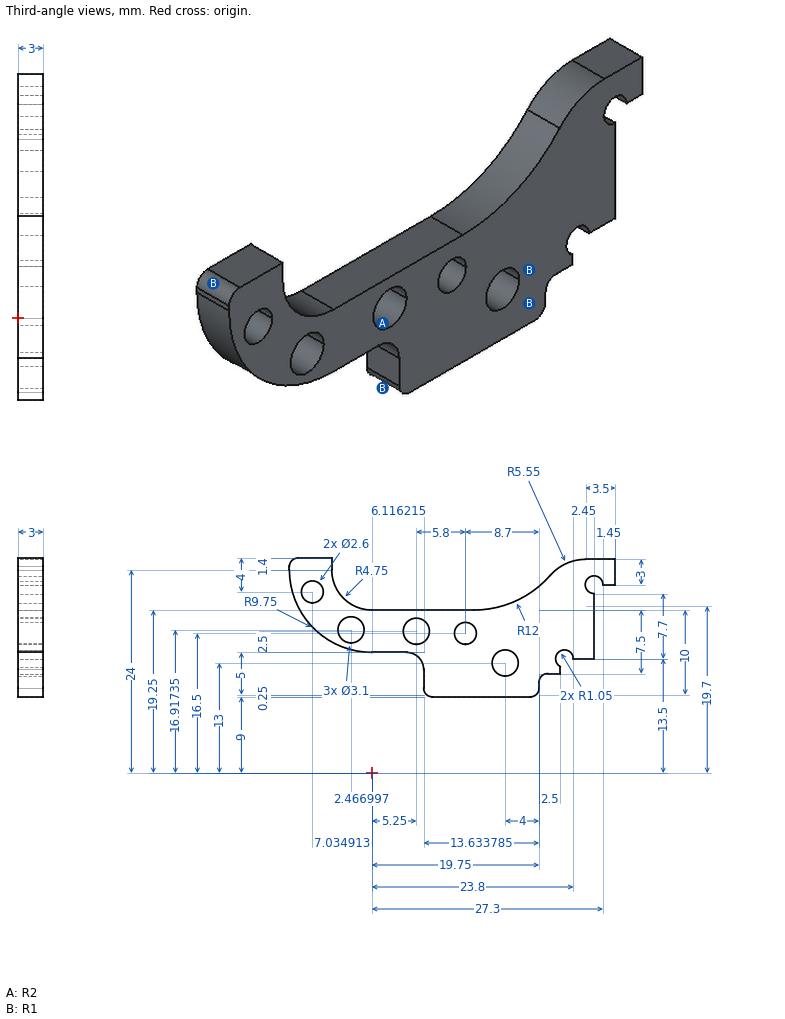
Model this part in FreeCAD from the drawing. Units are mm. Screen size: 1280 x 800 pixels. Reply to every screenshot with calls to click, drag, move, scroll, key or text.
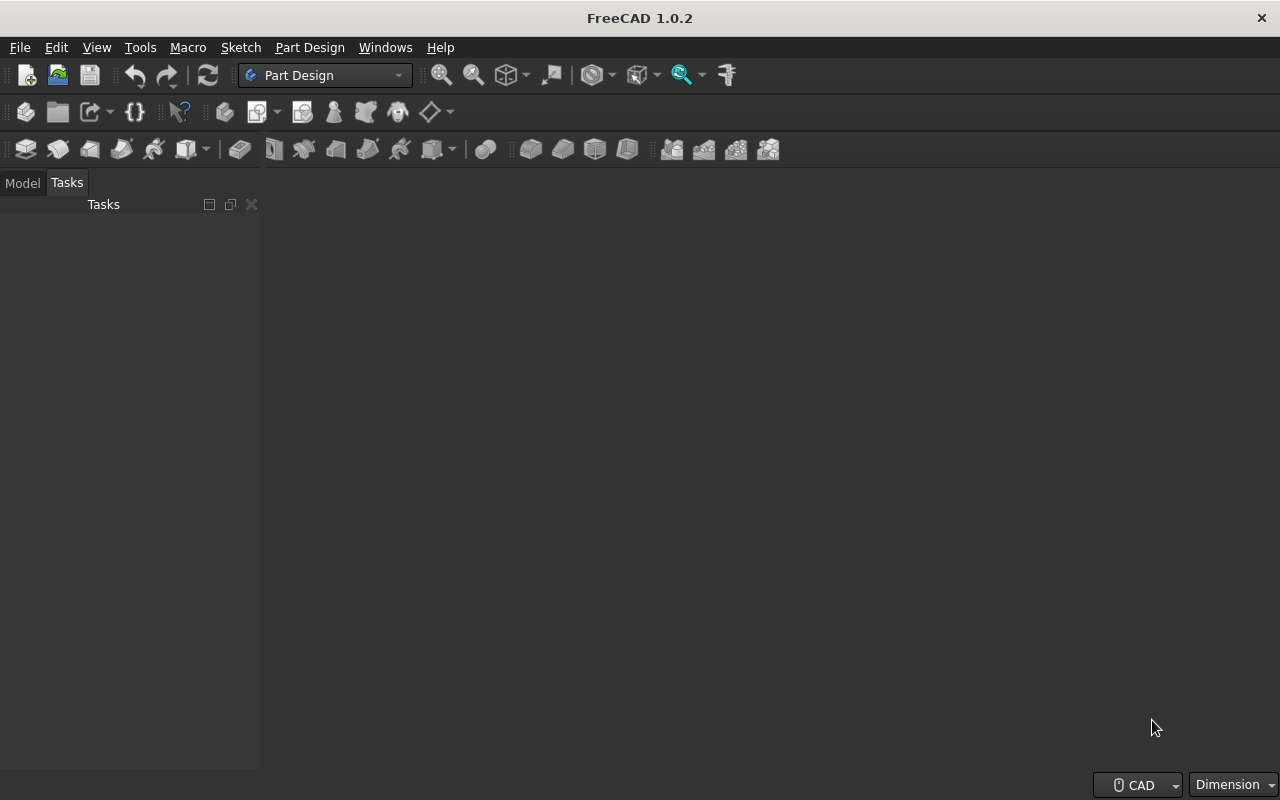
key(ctrl+n)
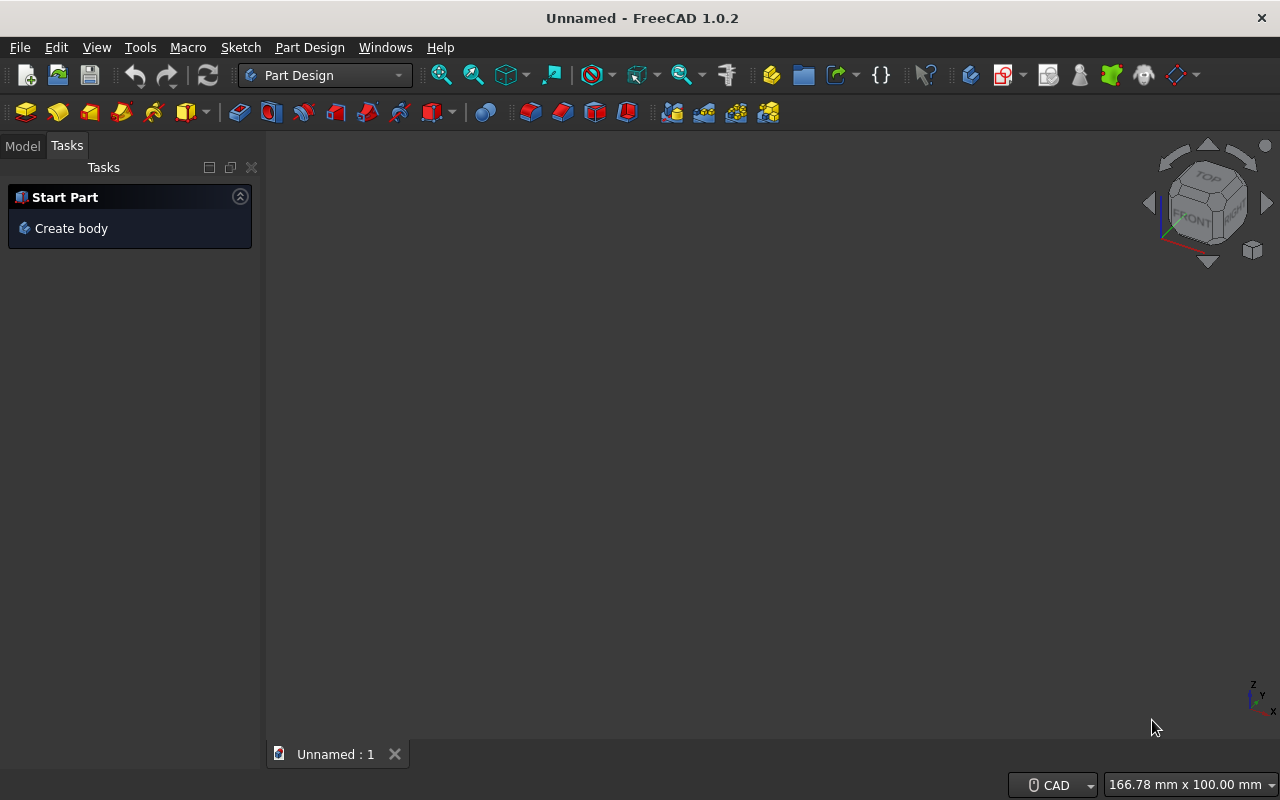
click(1004, 76)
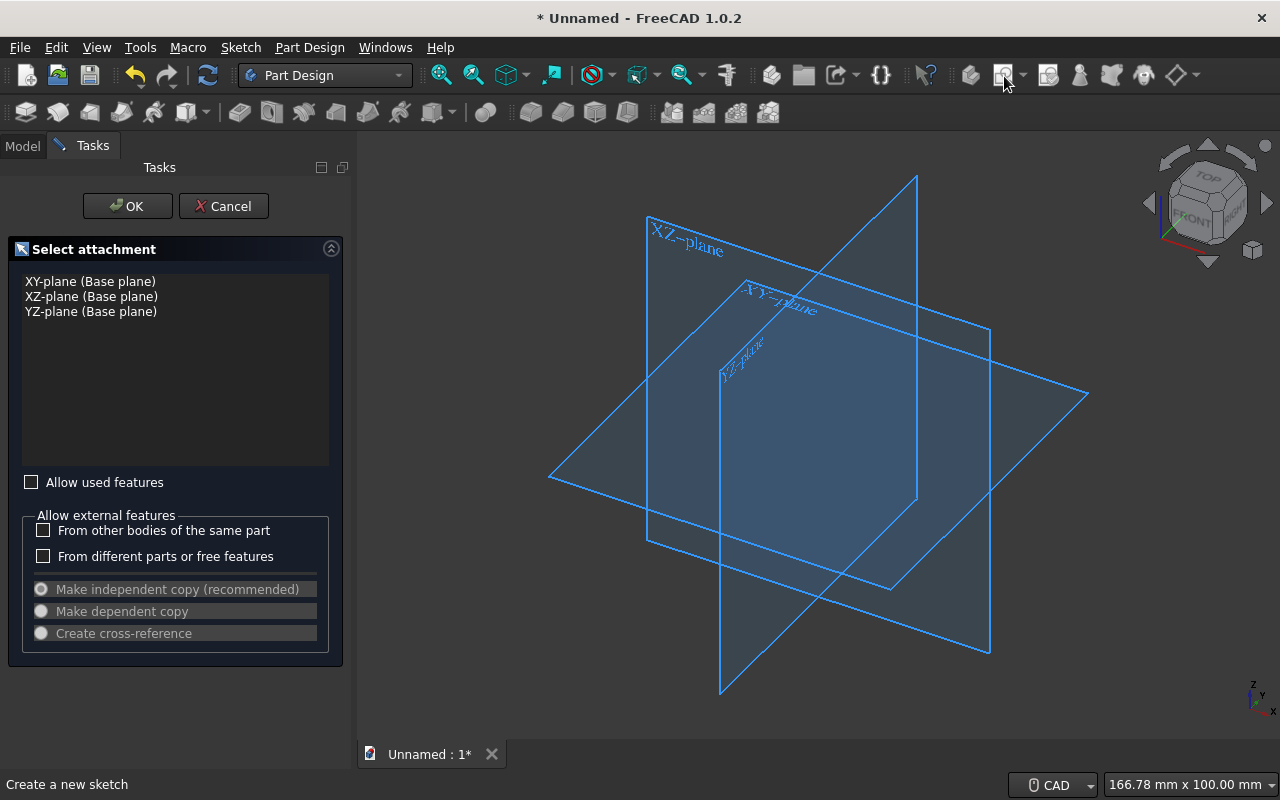
click(82, 312)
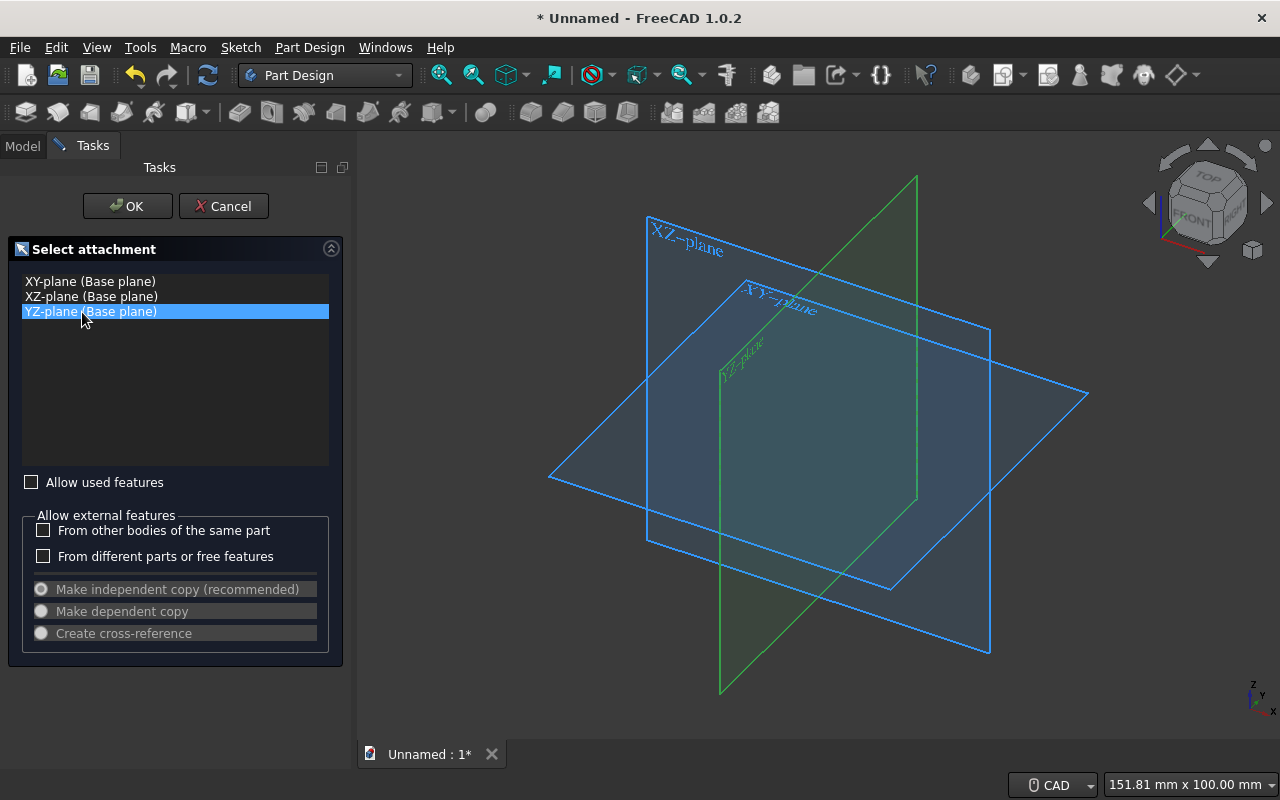
click(128, 206)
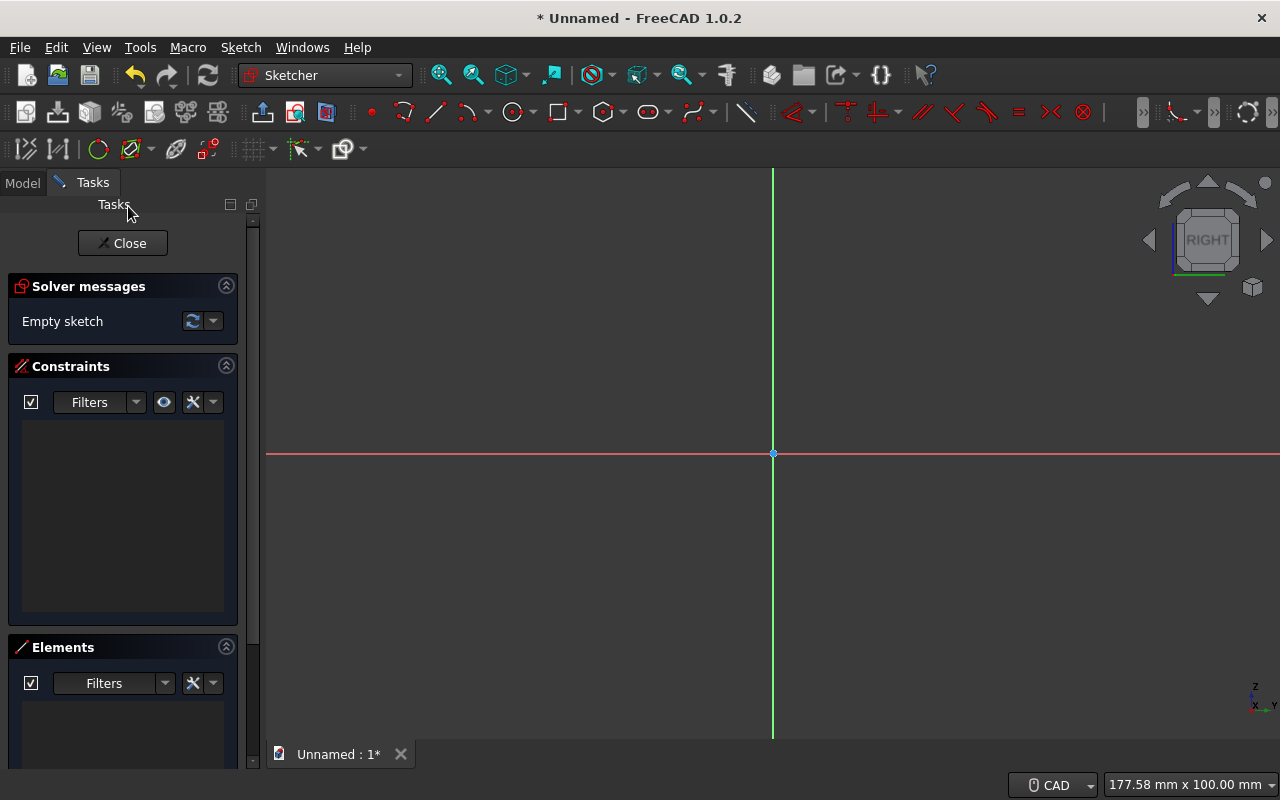
scroll(858, 339, up, 5)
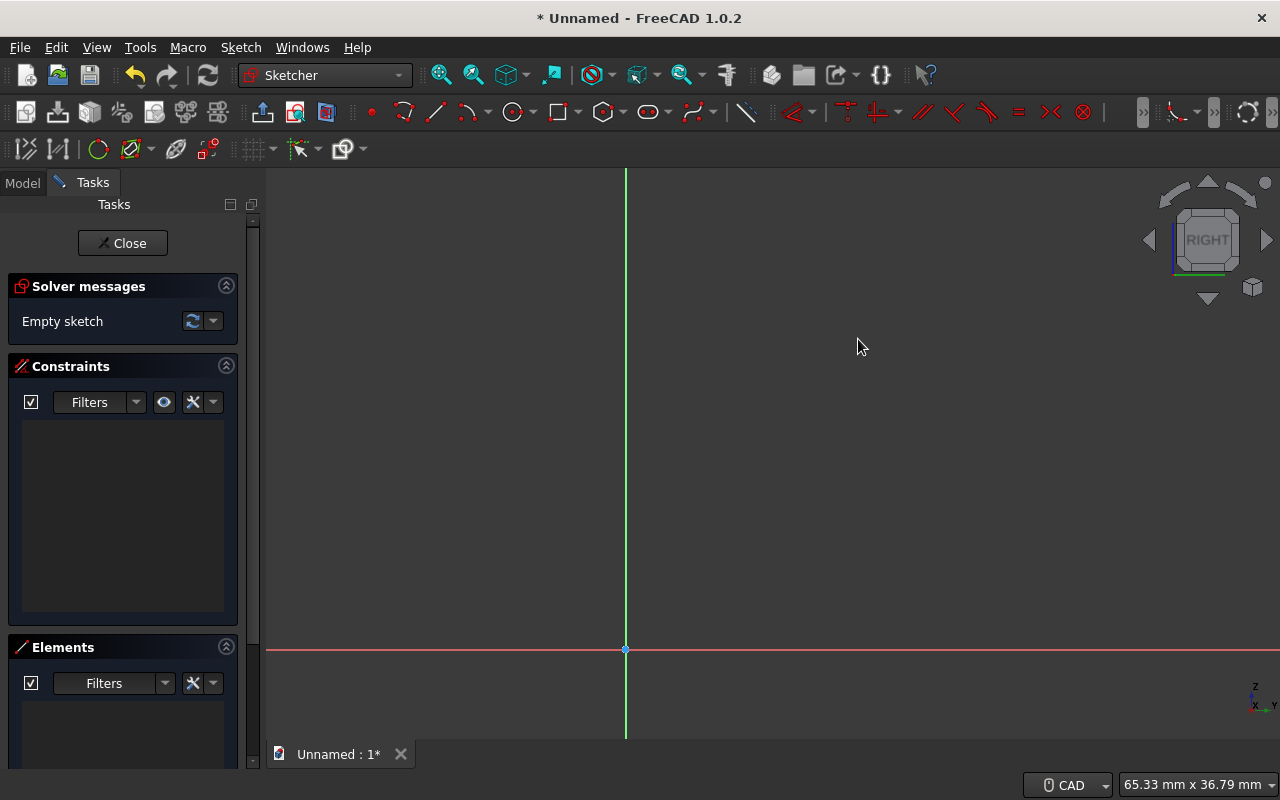
key(g)
key(m)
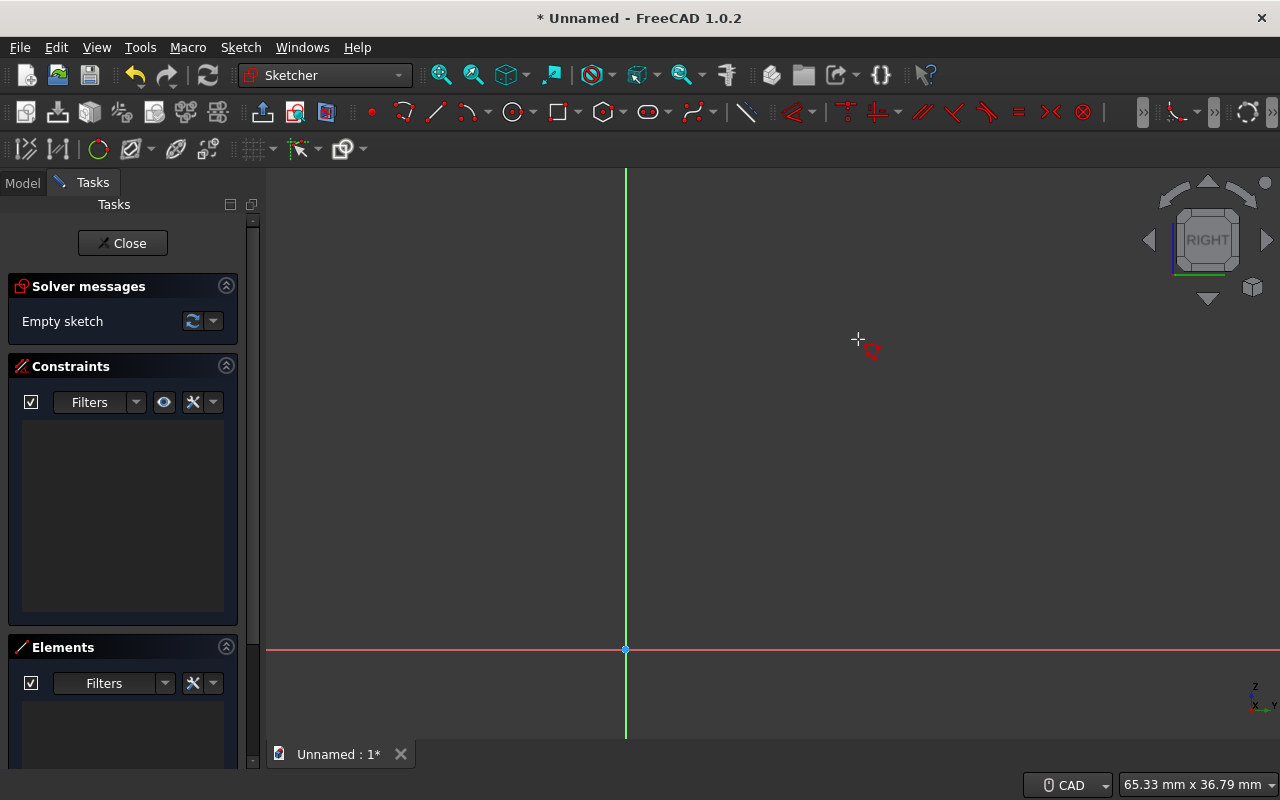
click(552, 277)
click(552, 255)
click(475, 255)
click(475, 277)
right_click(475, 277)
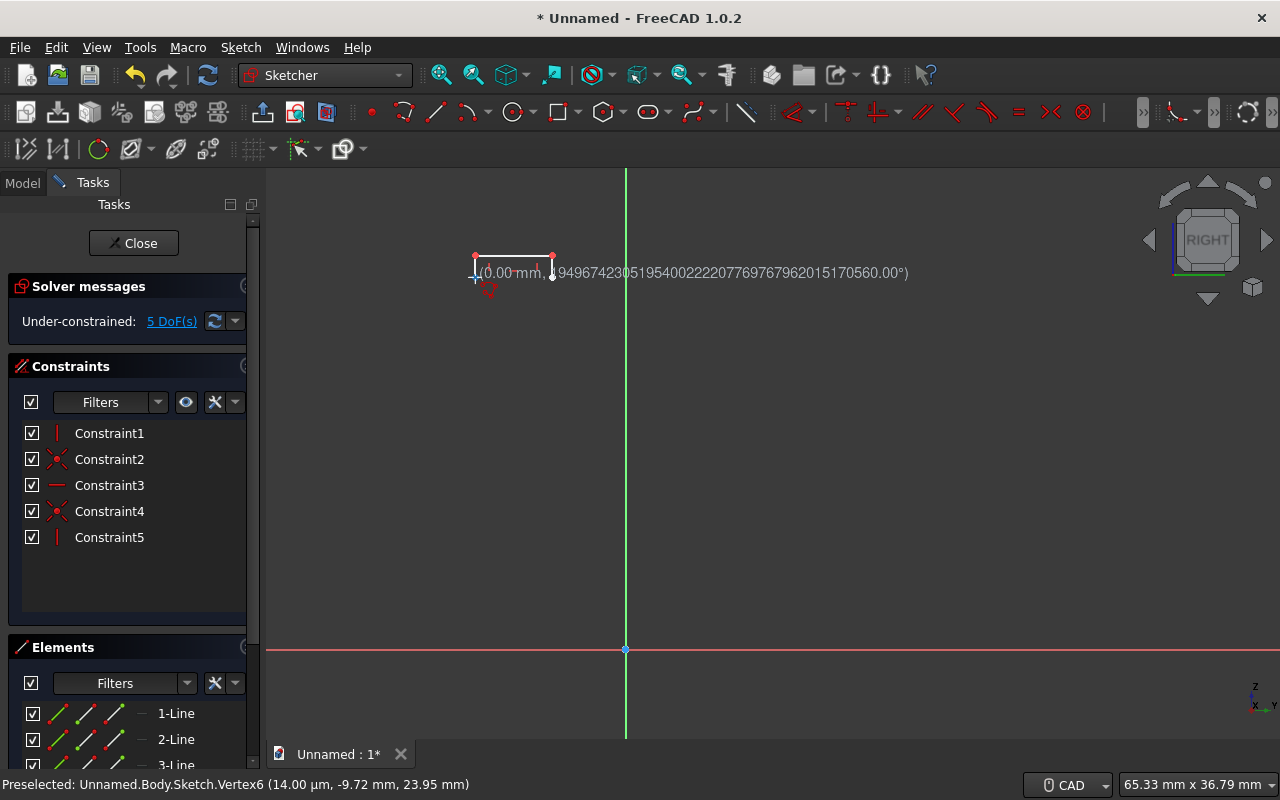
click(626, 429)
click(721, 429)
click(721, 506)
click(932, 506)
click(932, 351)
click(626, 351)
right_click(626, 351)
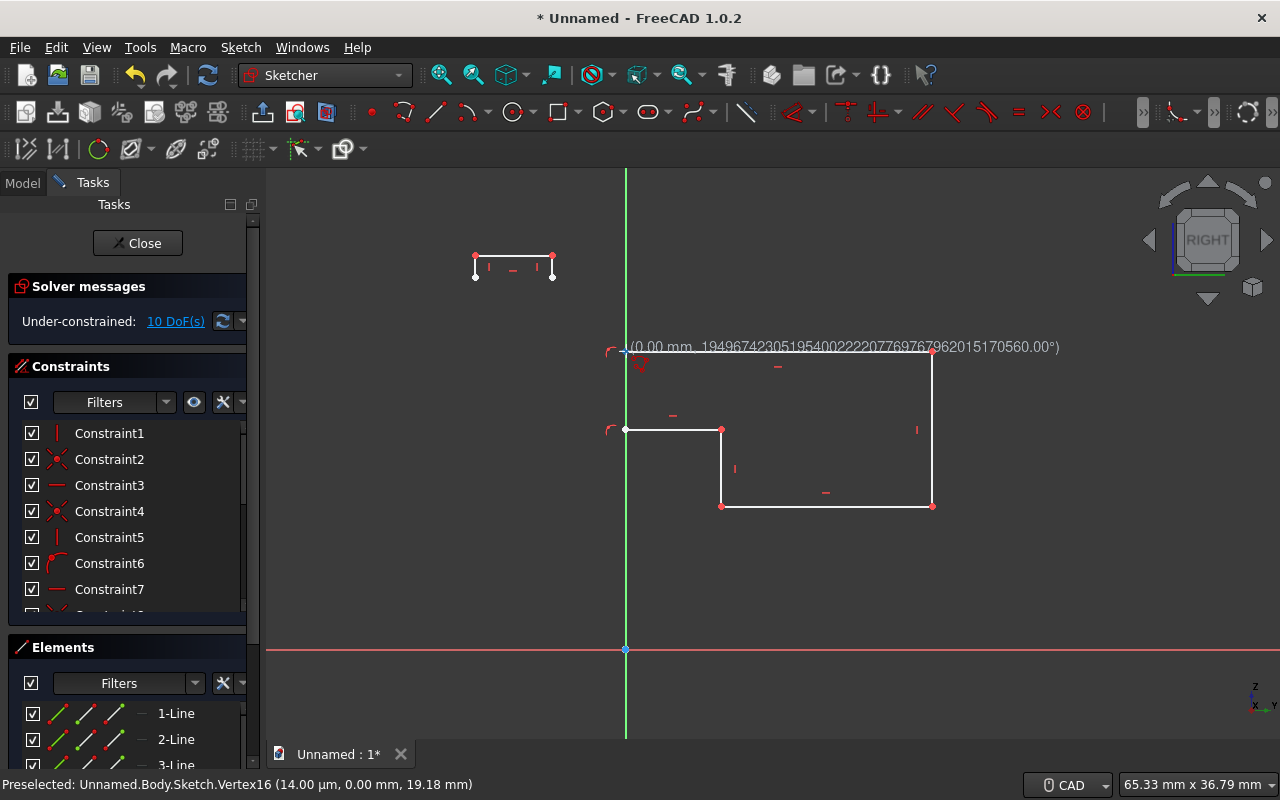
key(g)
key(3)
key(a)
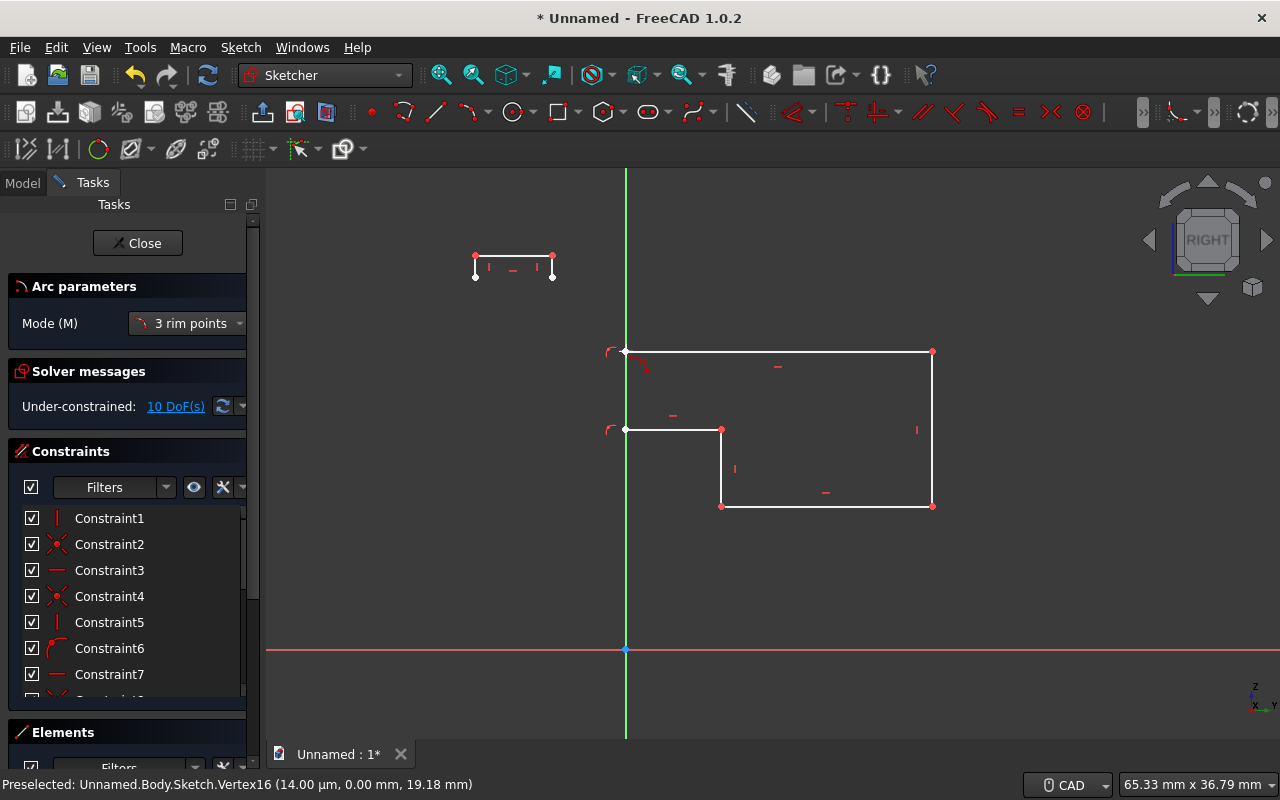
scroll(475, 277, up, 2)